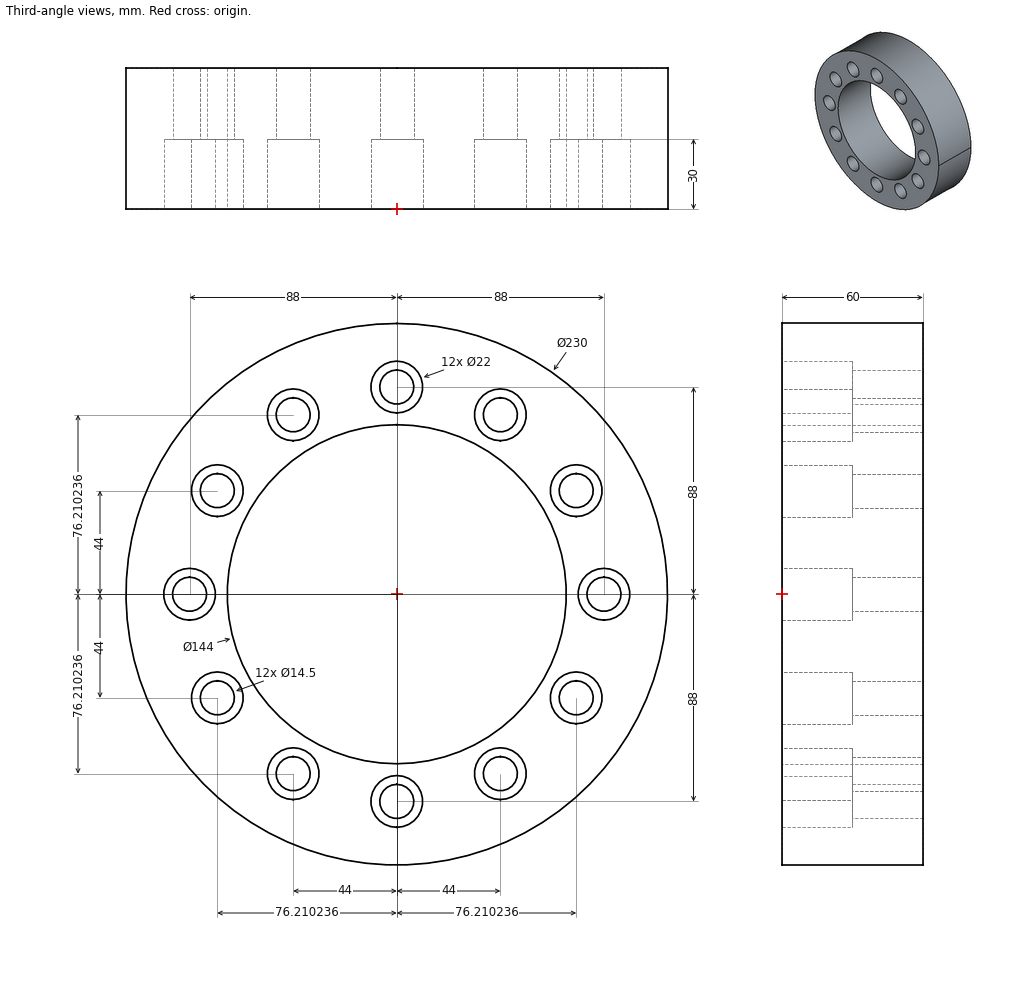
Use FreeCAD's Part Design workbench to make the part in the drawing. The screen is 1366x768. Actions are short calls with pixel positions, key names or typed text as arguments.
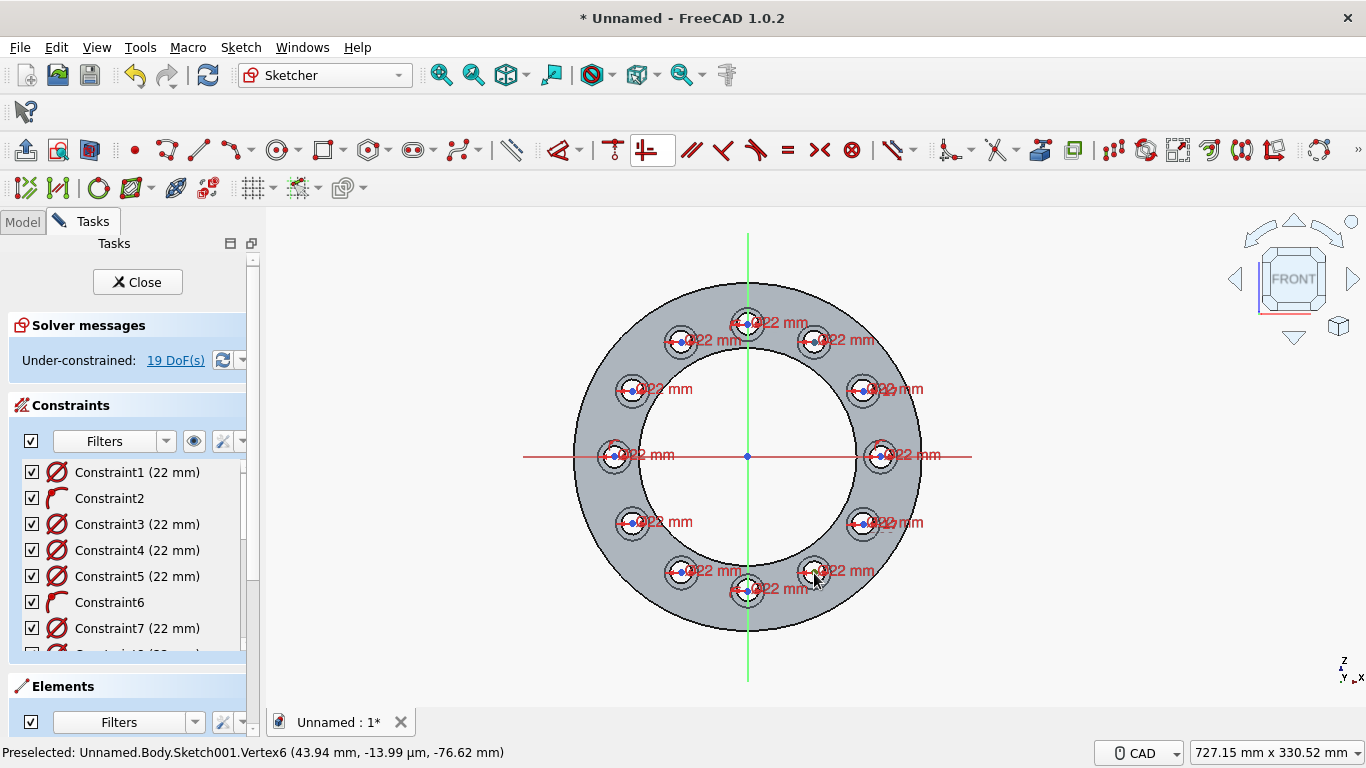
key(v)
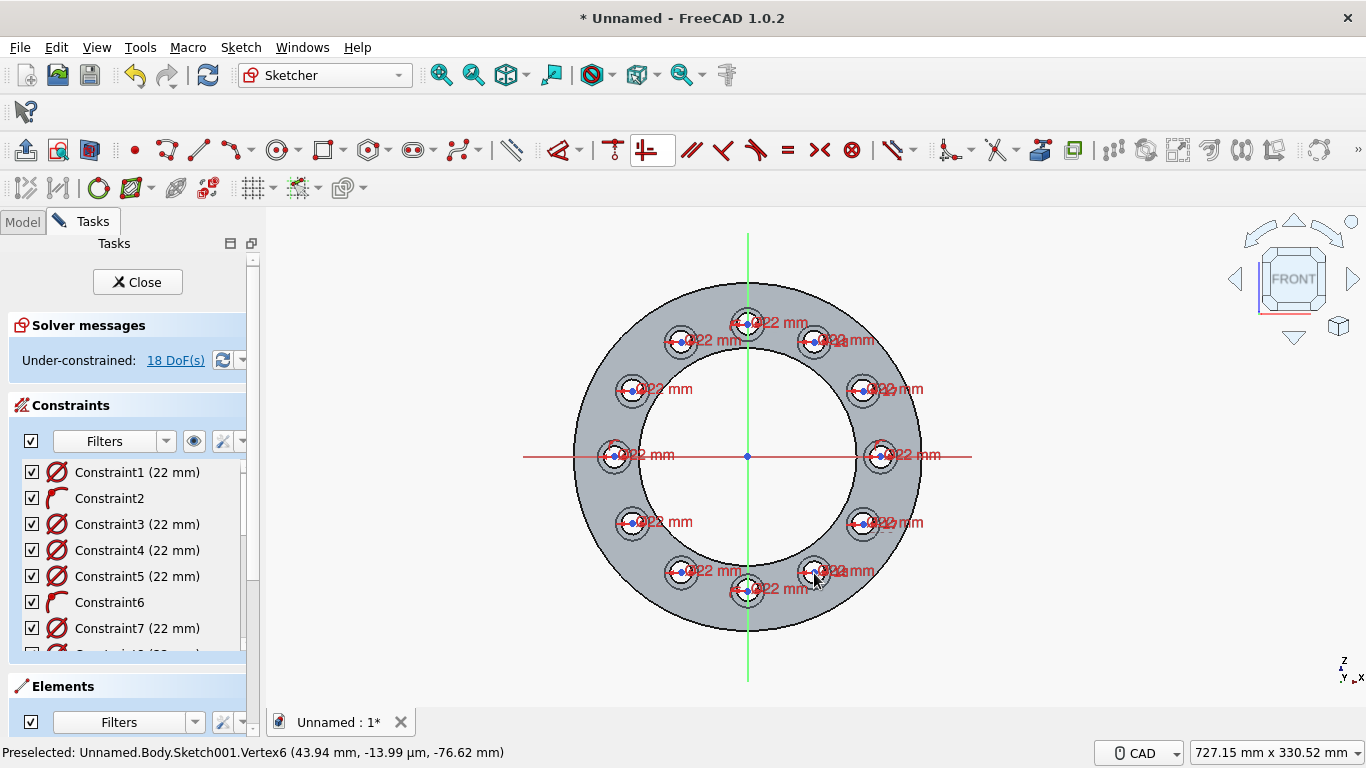
click(814, 573)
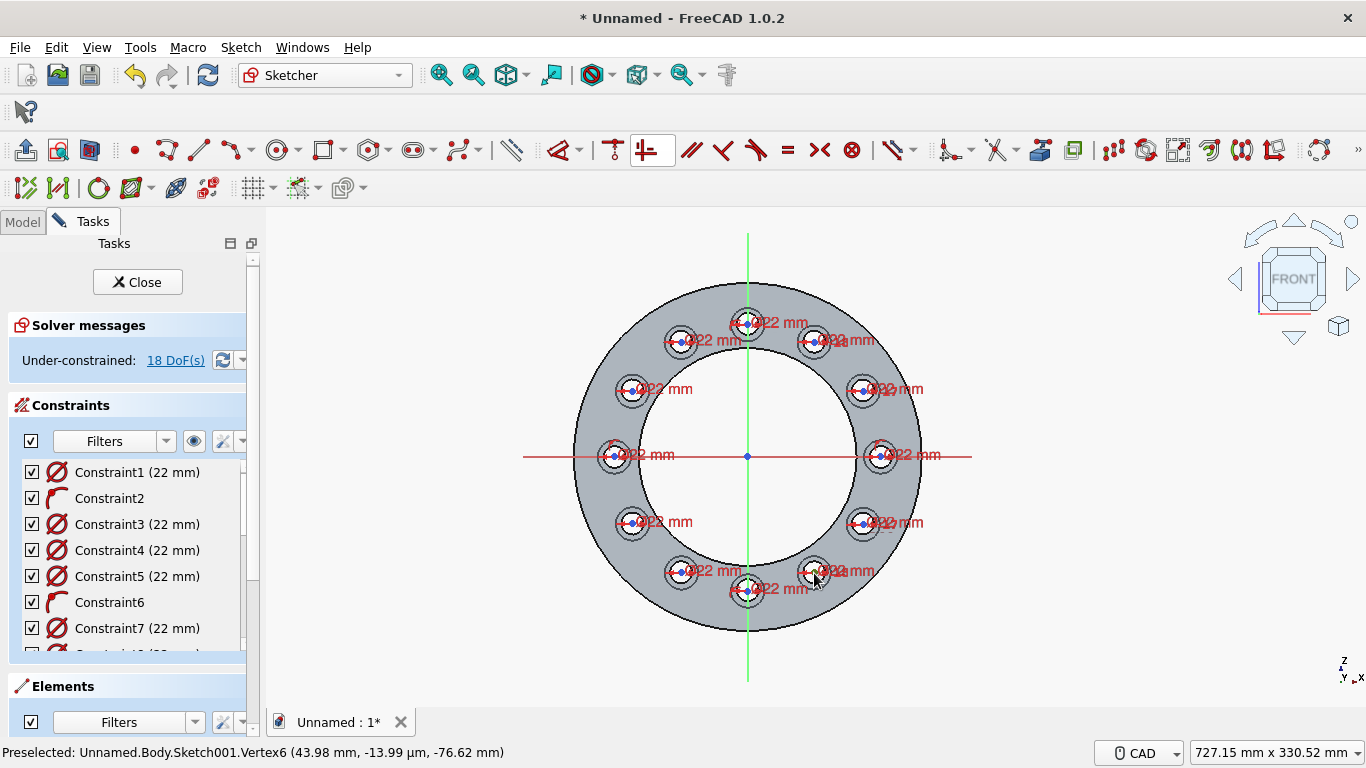
click(681, 573)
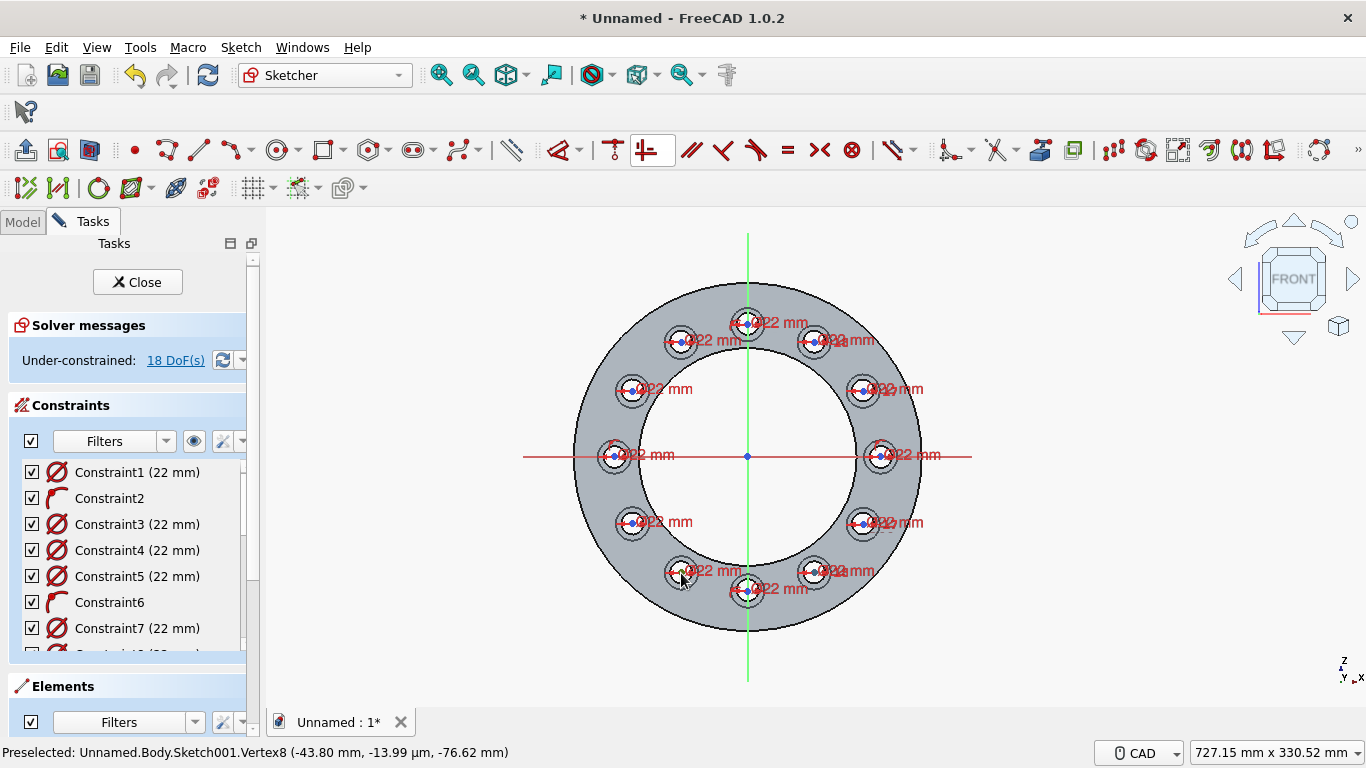
key(h)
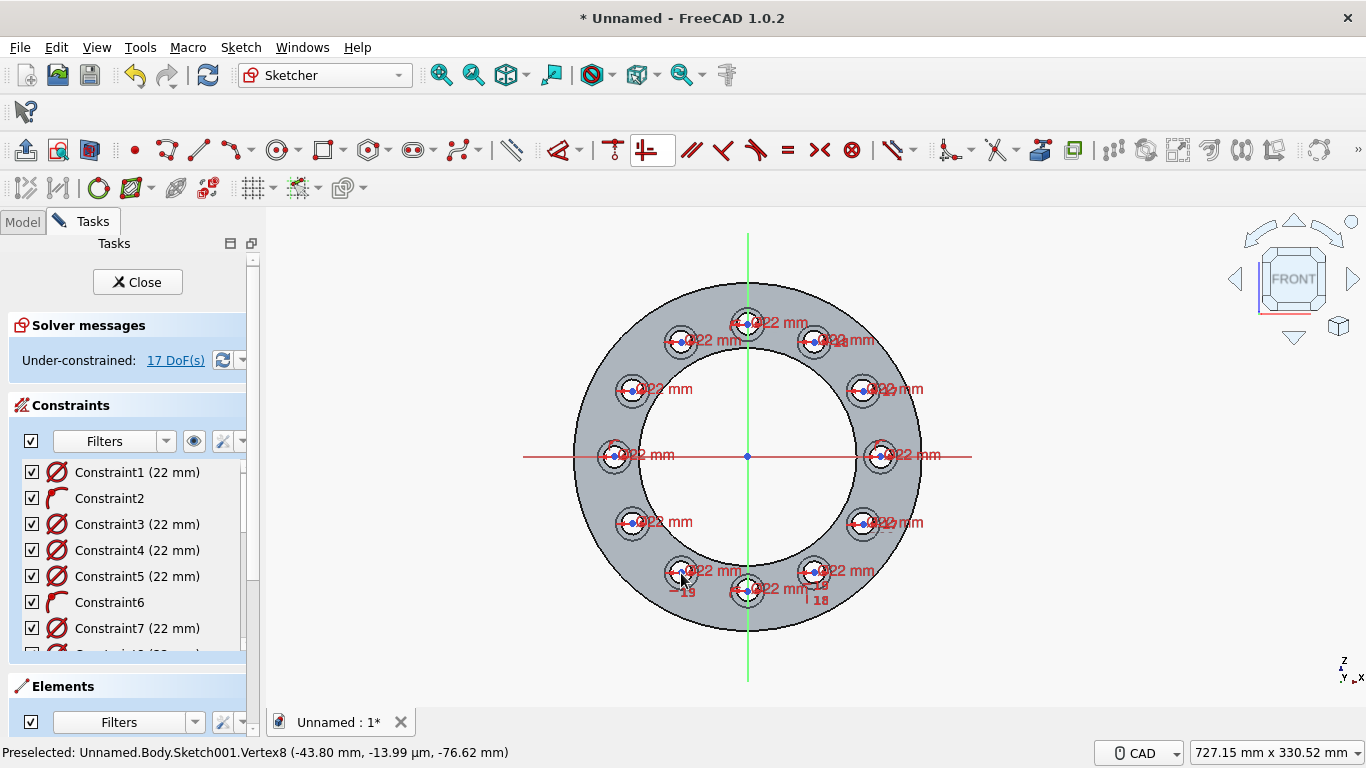
click(863, 525)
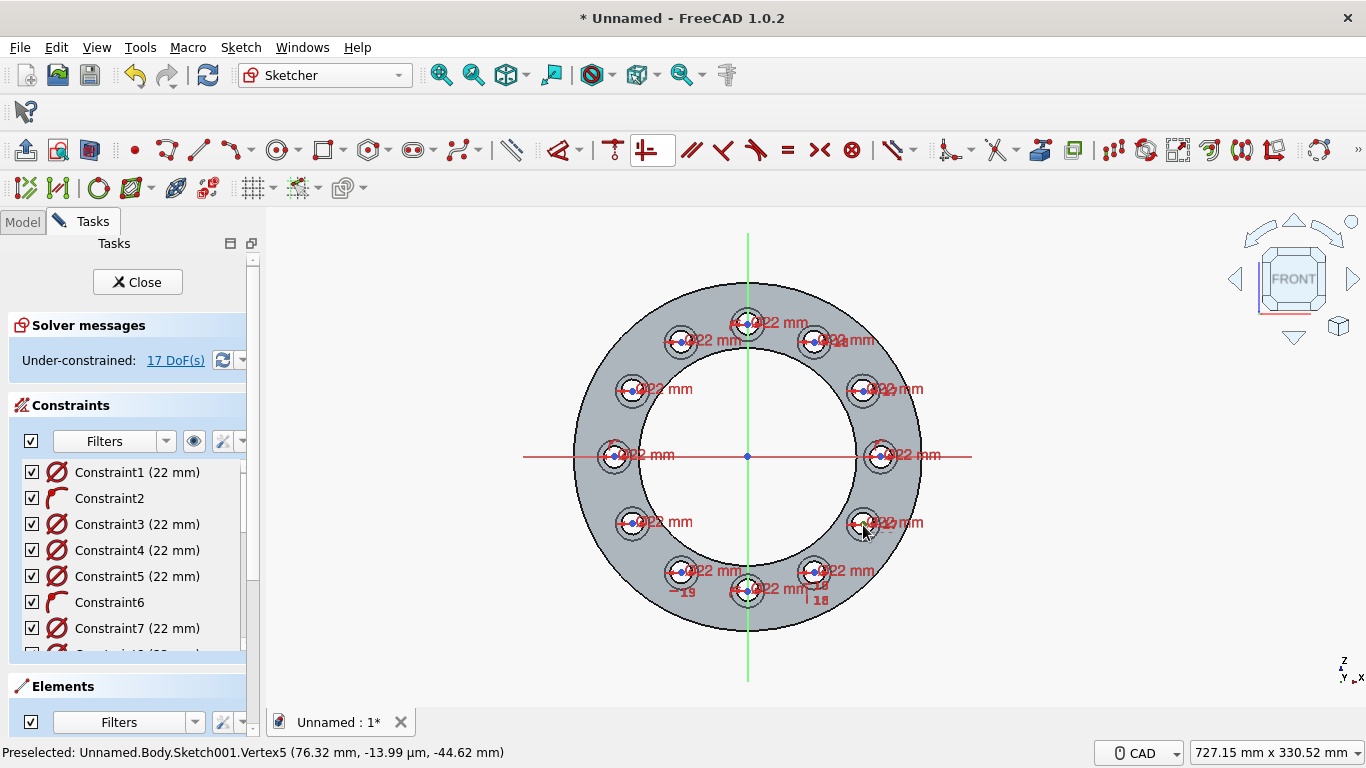
click(633, 524)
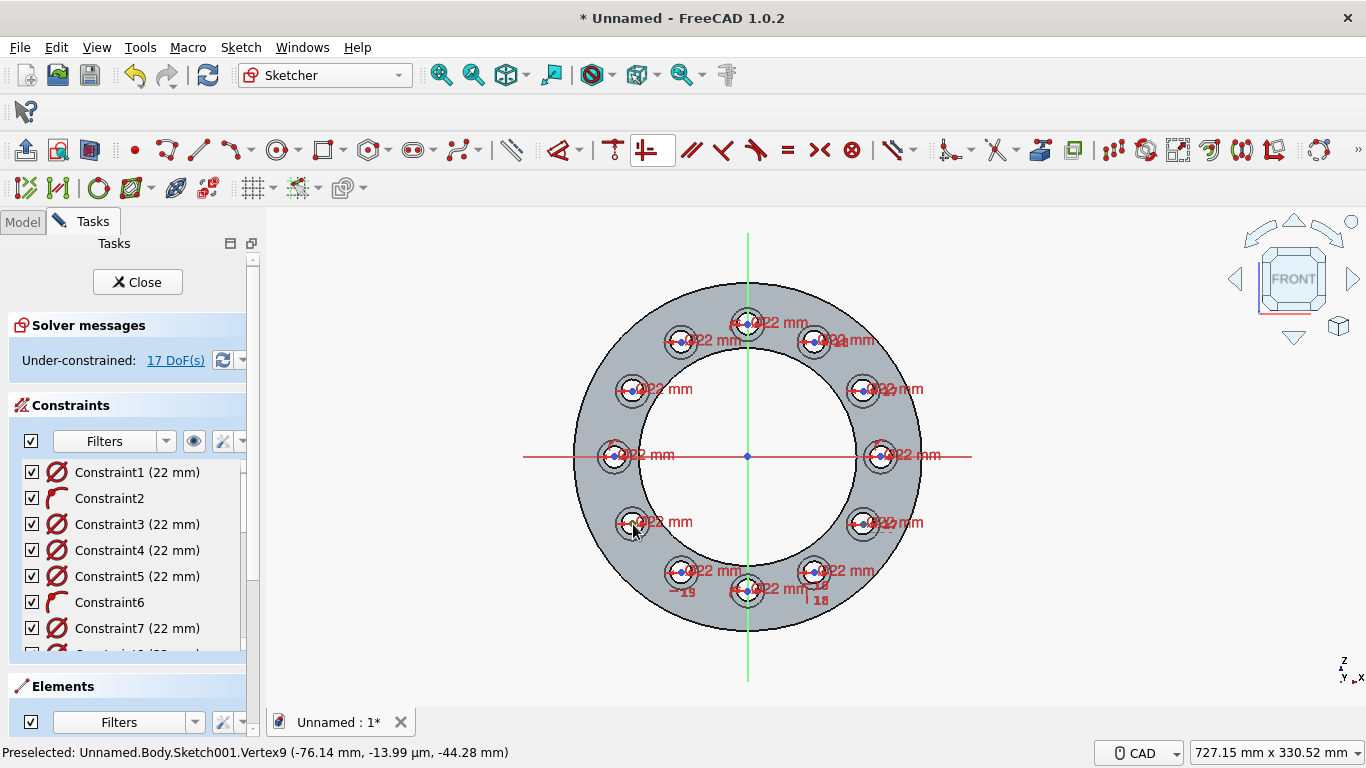
key(h)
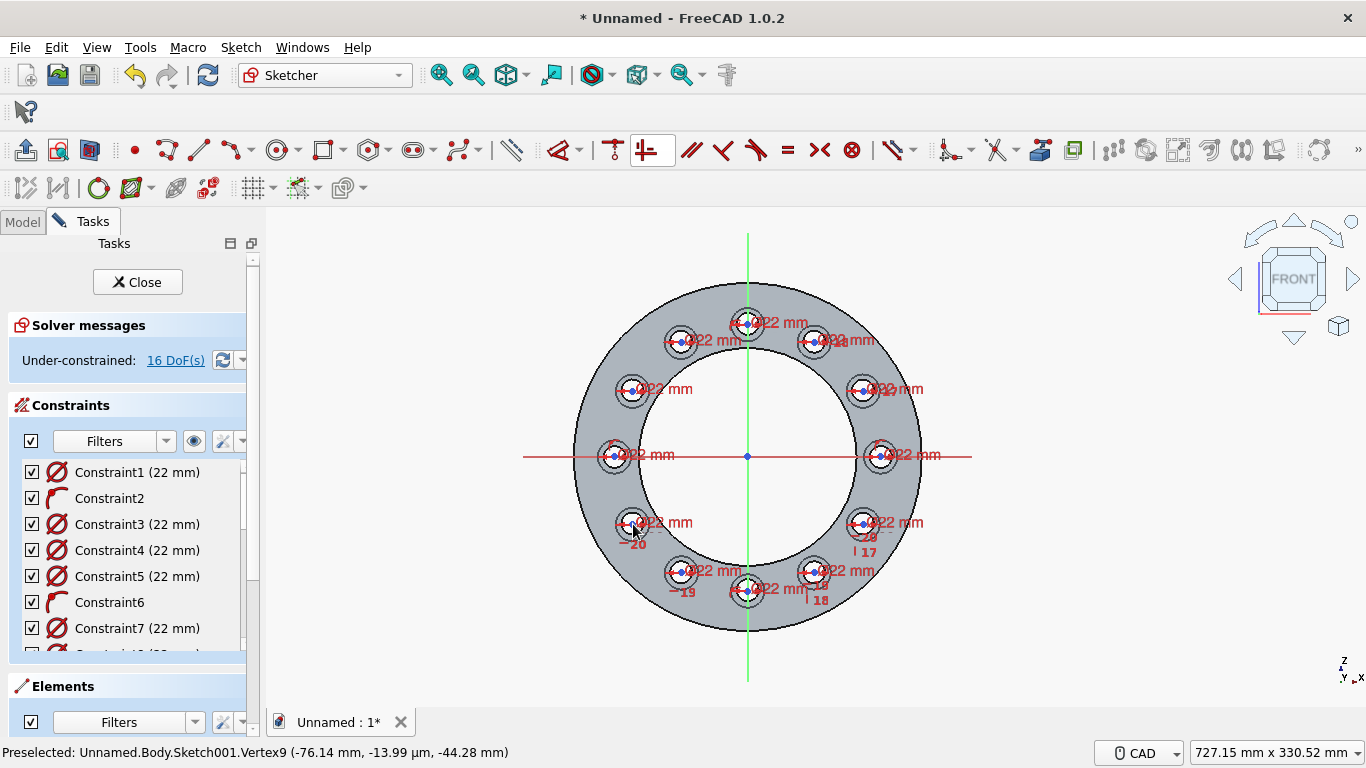
click(633, 525)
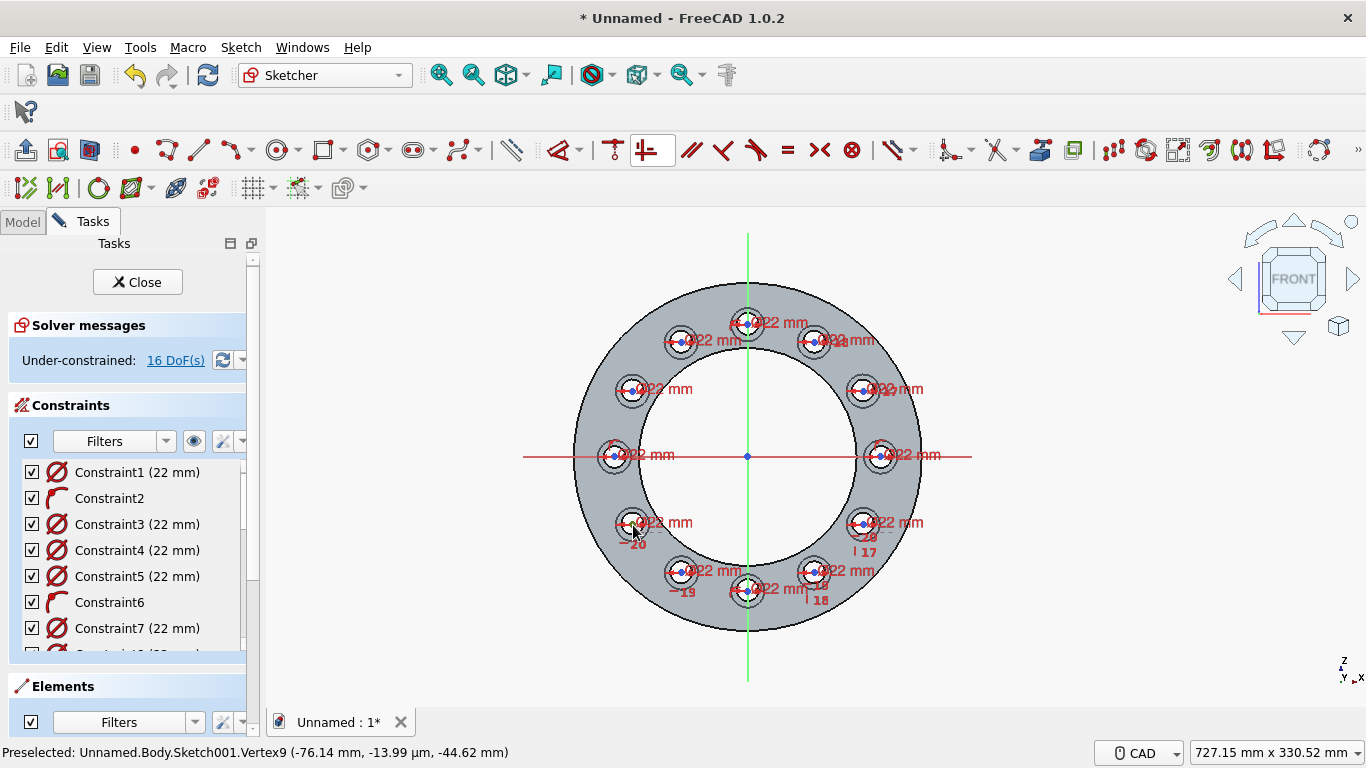
click(633, 391)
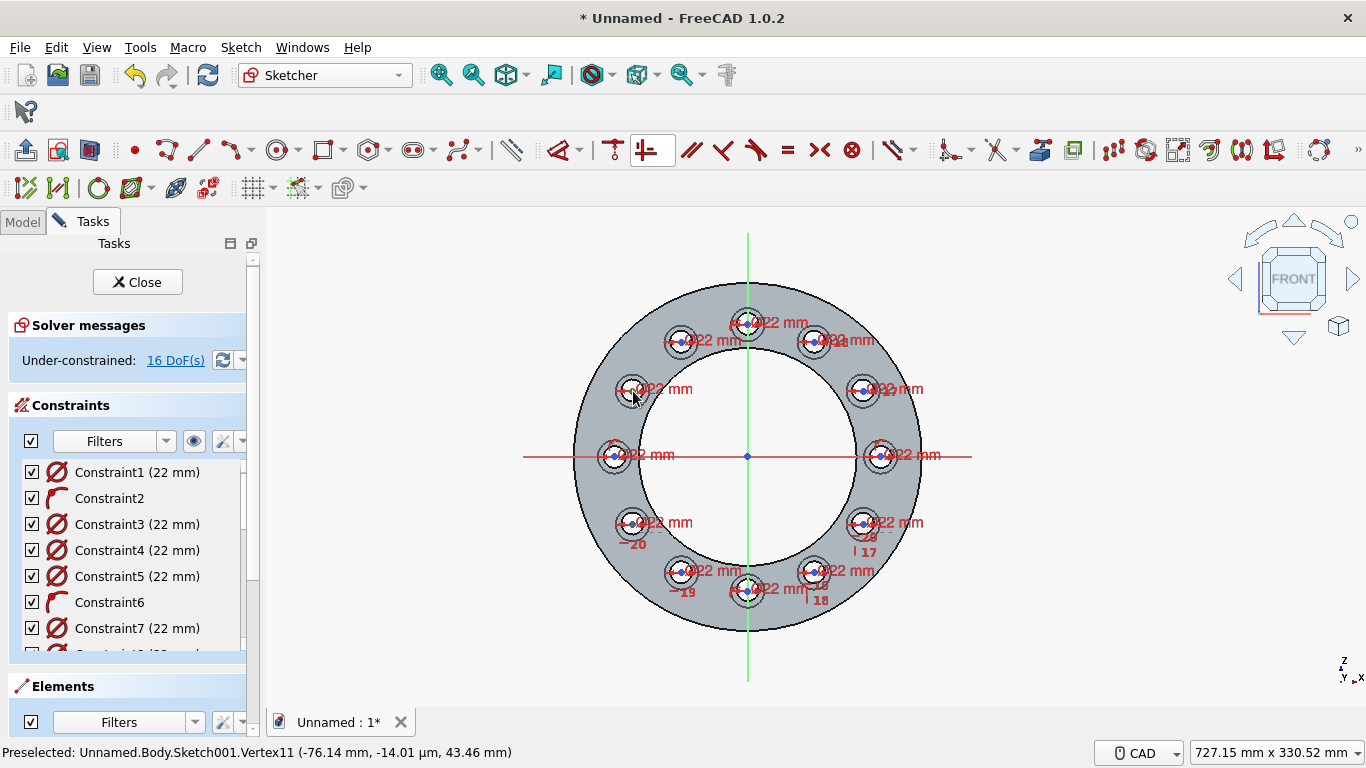
key(v)